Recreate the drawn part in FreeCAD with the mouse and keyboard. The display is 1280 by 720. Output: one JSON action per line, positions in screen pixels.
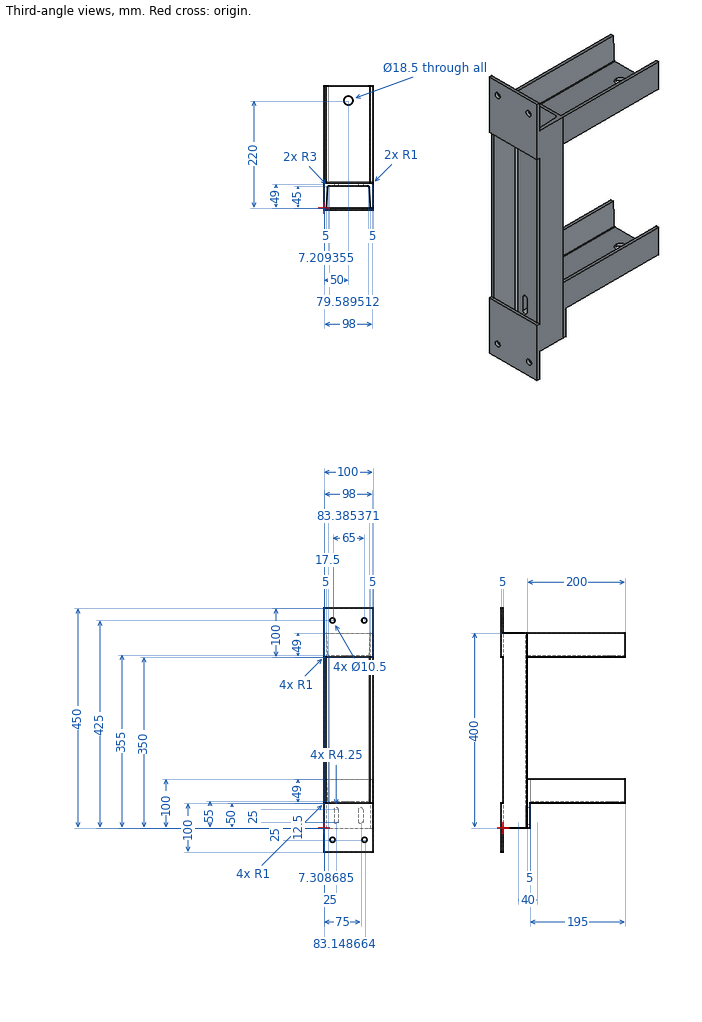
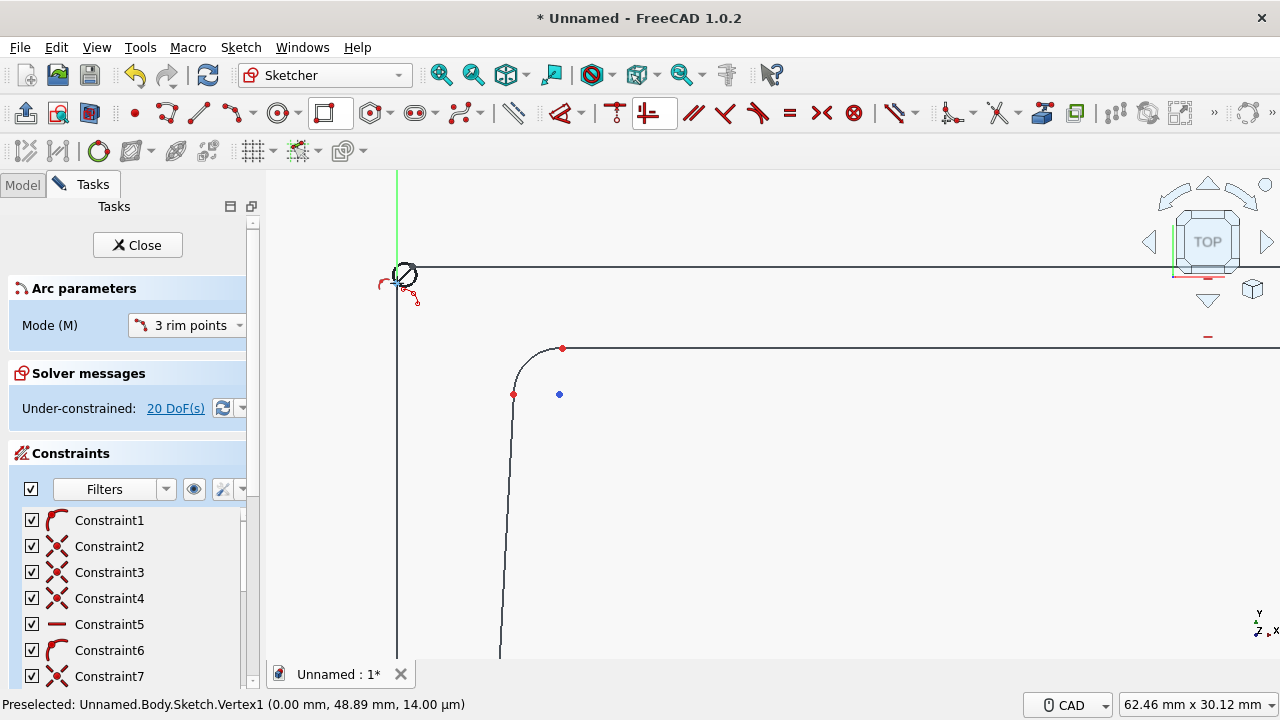
{"action": "scroll", "coordinate": [401, 270], "scroll_direction": "up", "scroll_amount": 7}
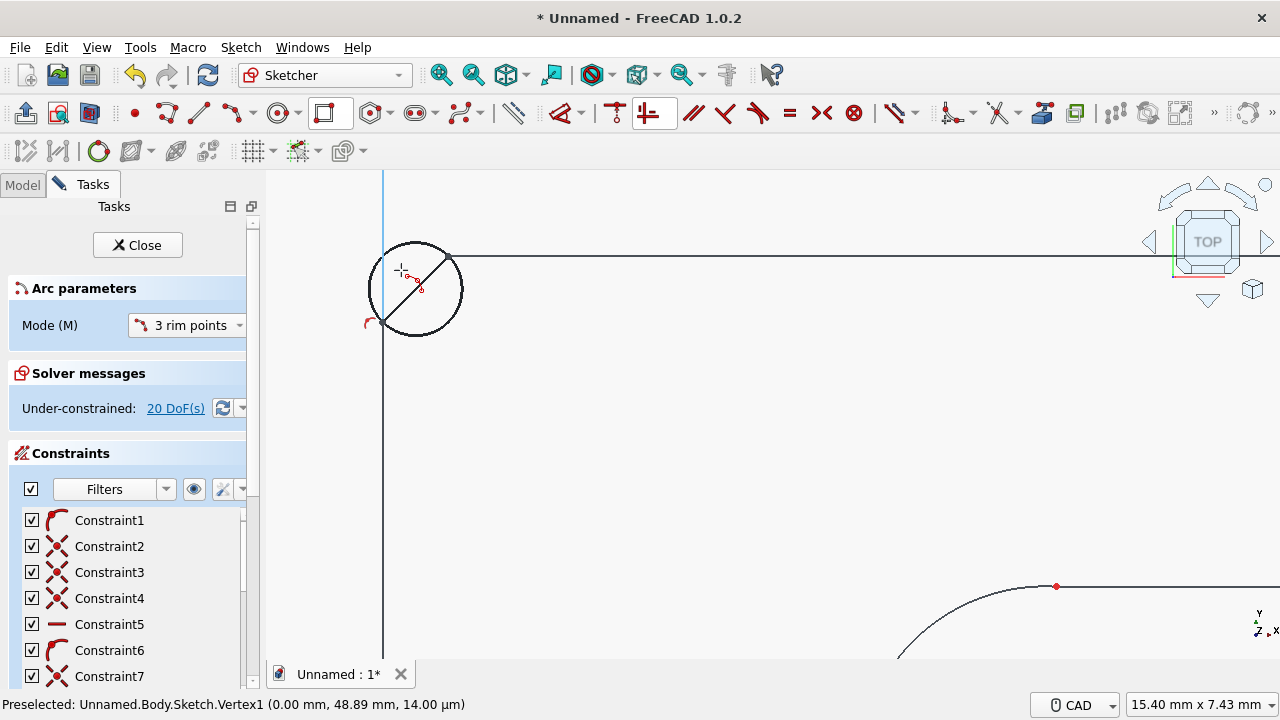
{"action": "left_click", "coordinate": [402, 268]}
{"action": "key", "text": "Escape"}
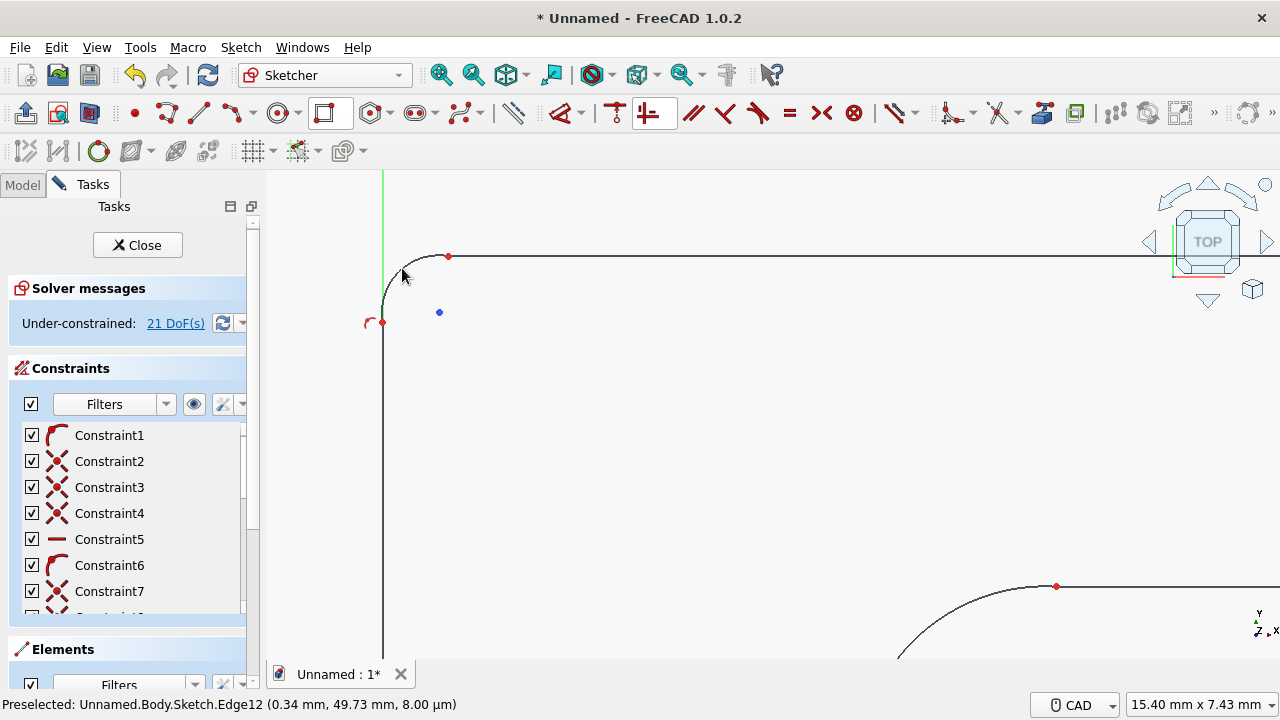
{"action": "scroll", "coordinate": [408, 267], "scroll_direction": "down", "scroll_amount": 12}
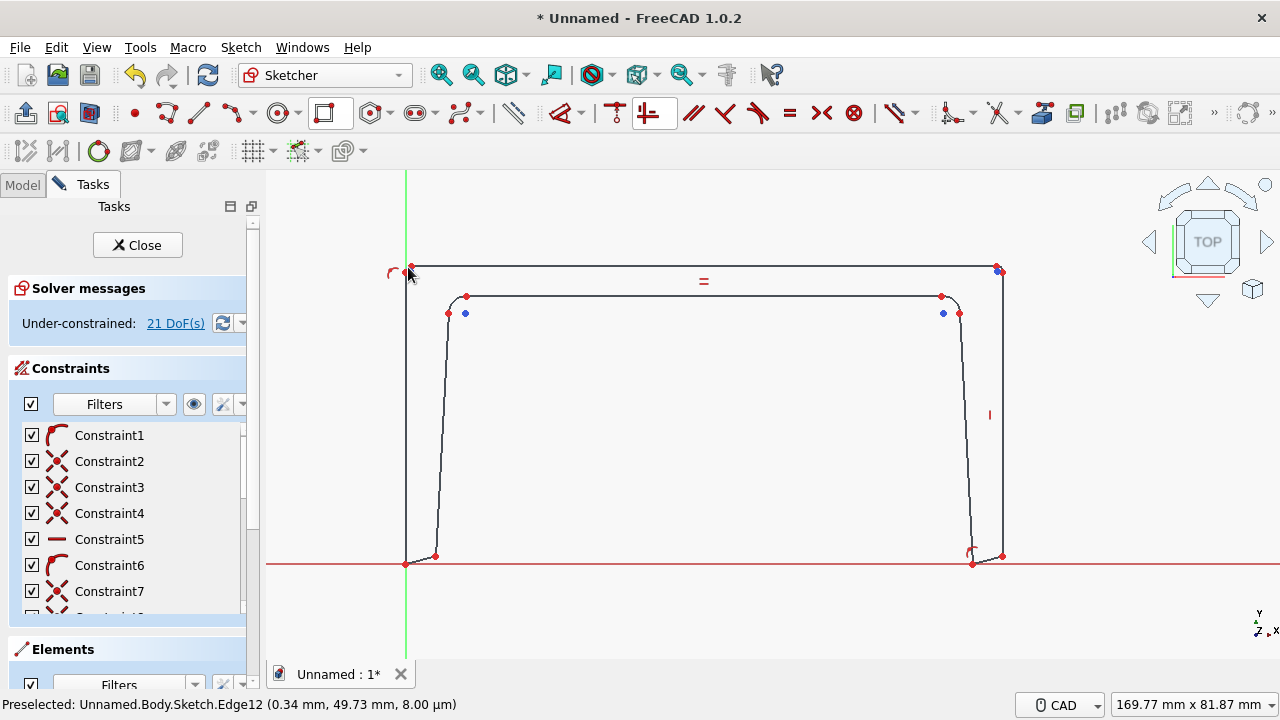
{"action": "left_click", "coordinate": [406, 360]}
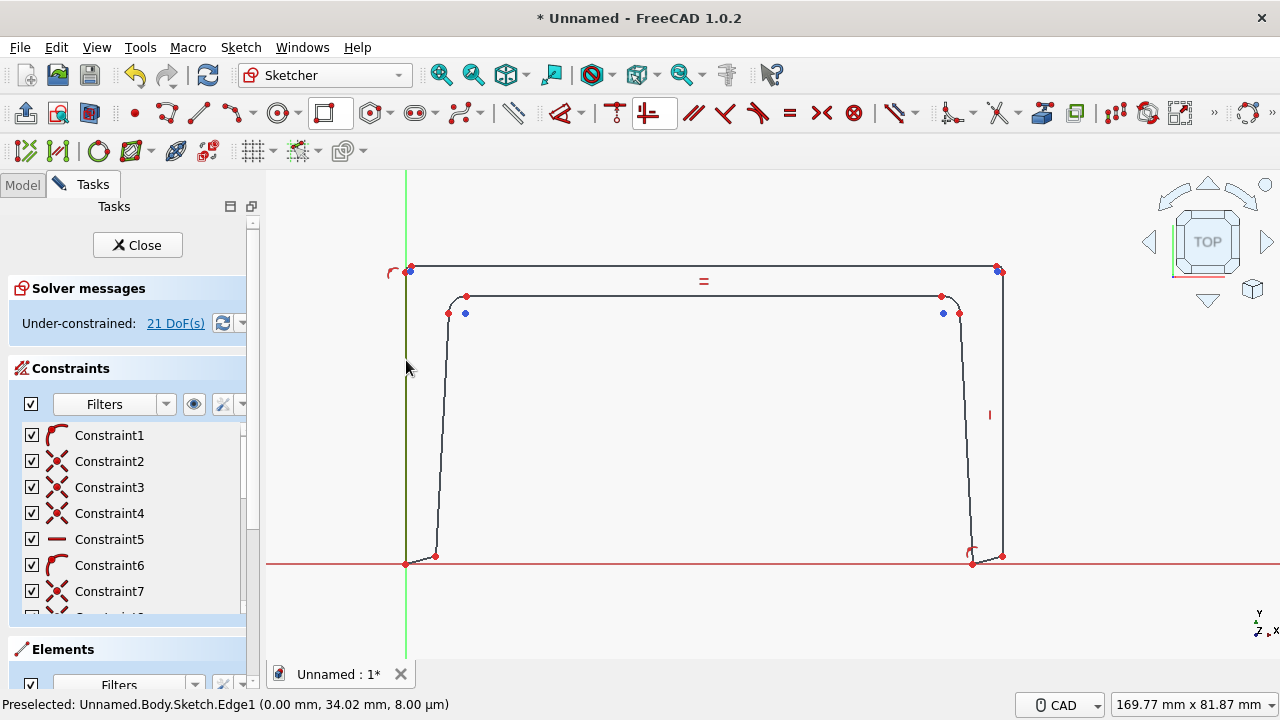
{"action": "scroll", "coordinate": [407, 268], "scroll_direction": "up", "scroll_amount": 6}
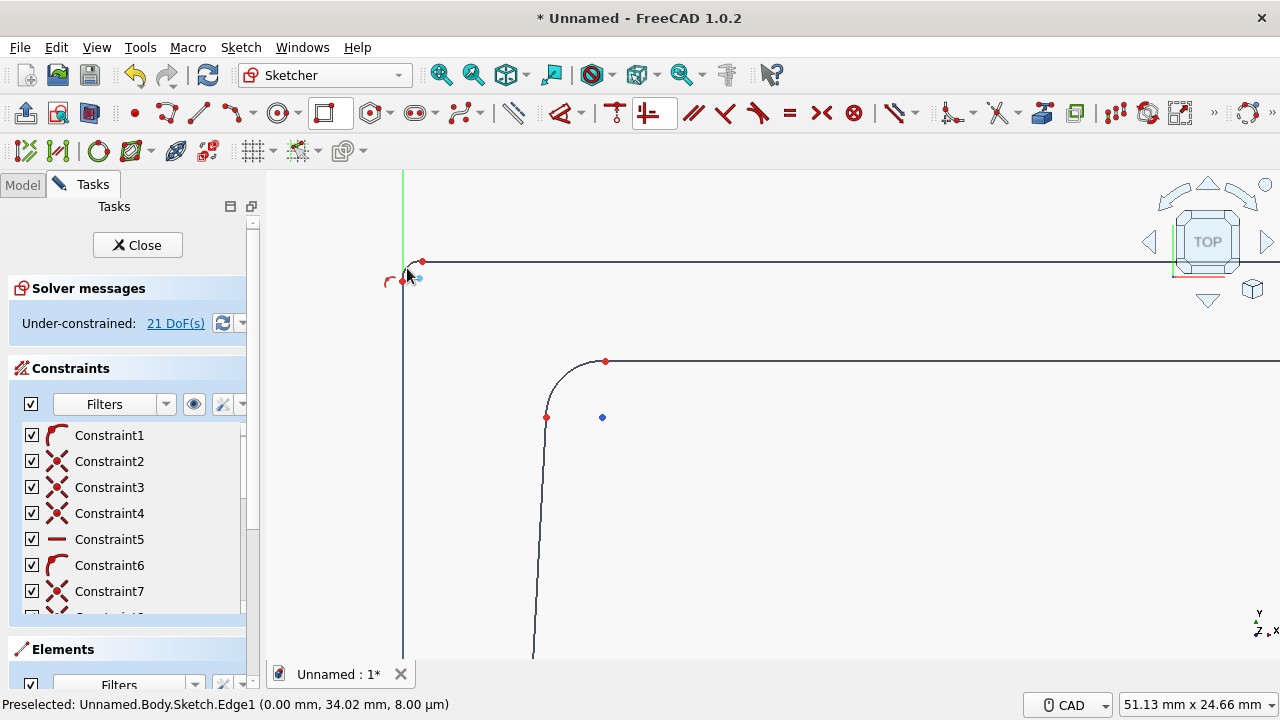
{"action": "left_click", "coordinate": [408, 266]}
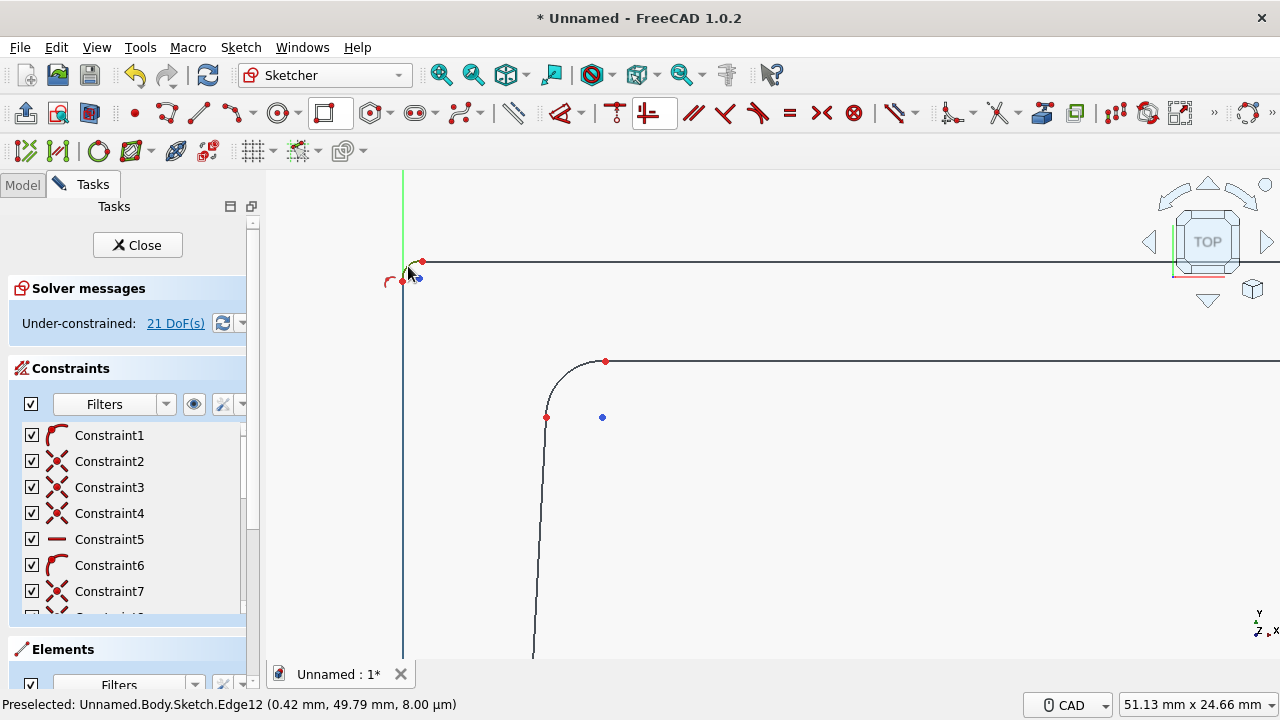
{"action": "left_click", "coordinate": [758, 114]}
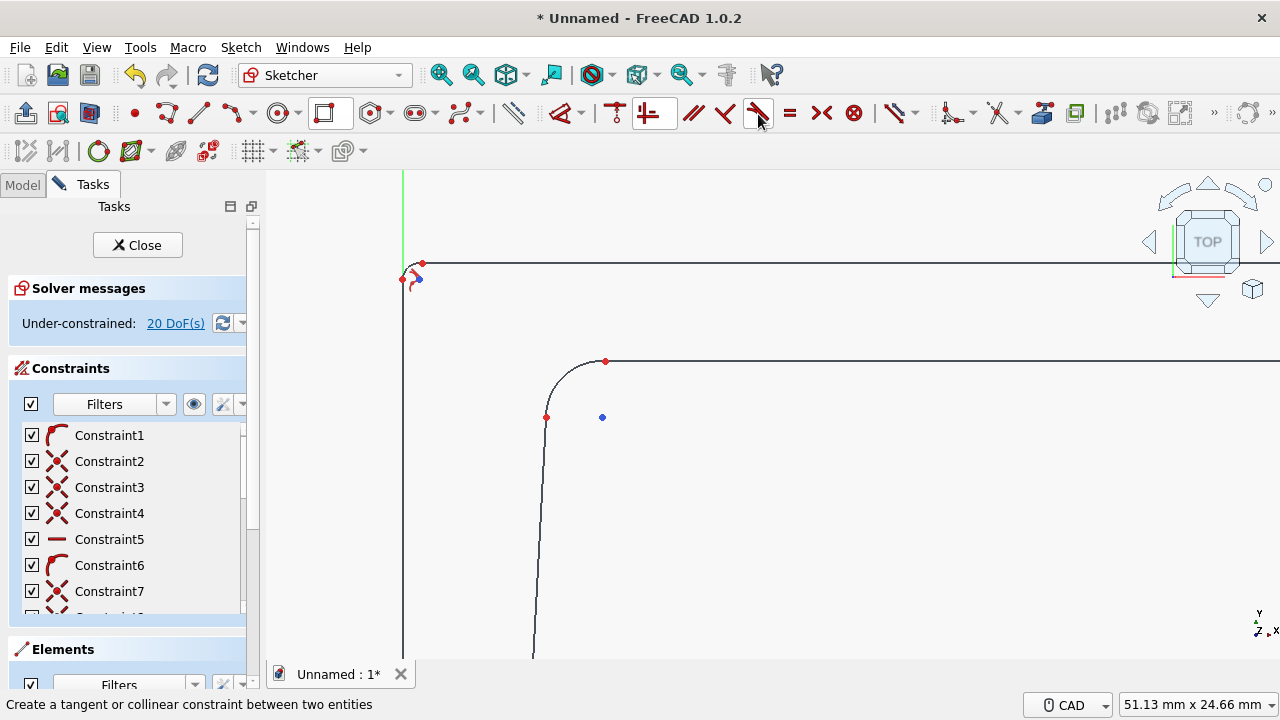
{"action": "left_click", "coordinate": [537, 579]}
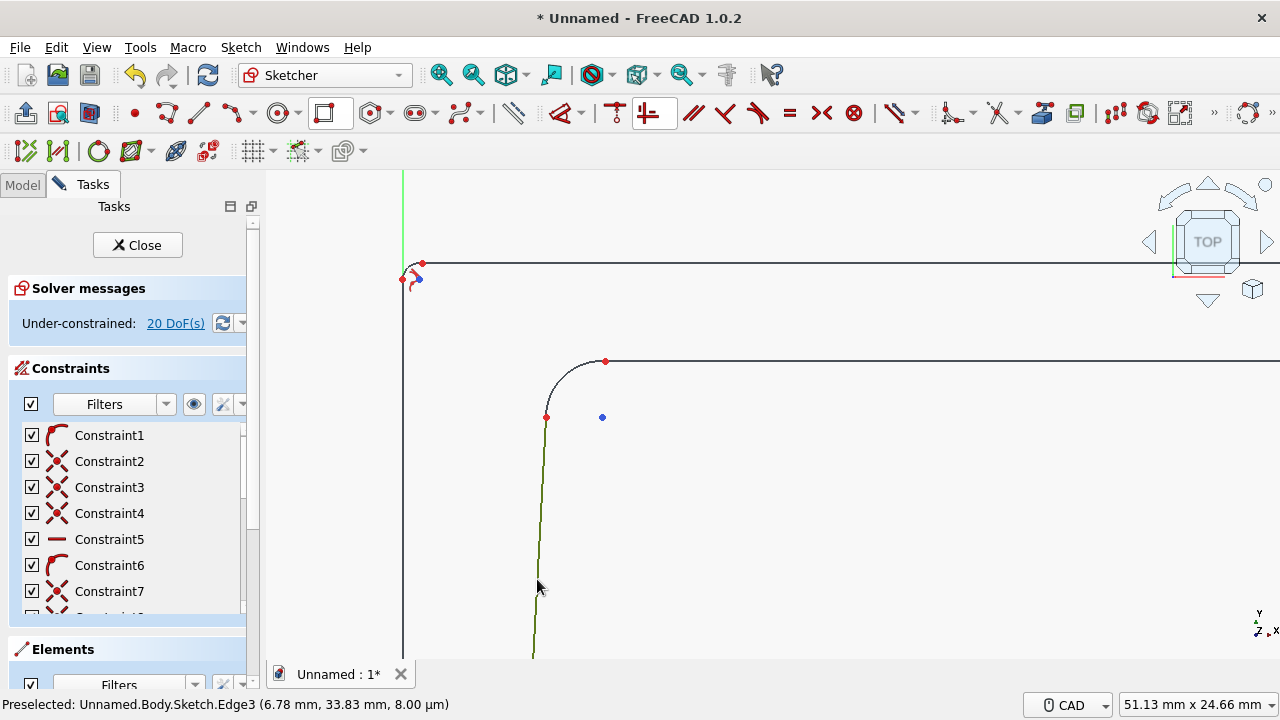
{"action": "left_click", "coordinate": [579, 366]}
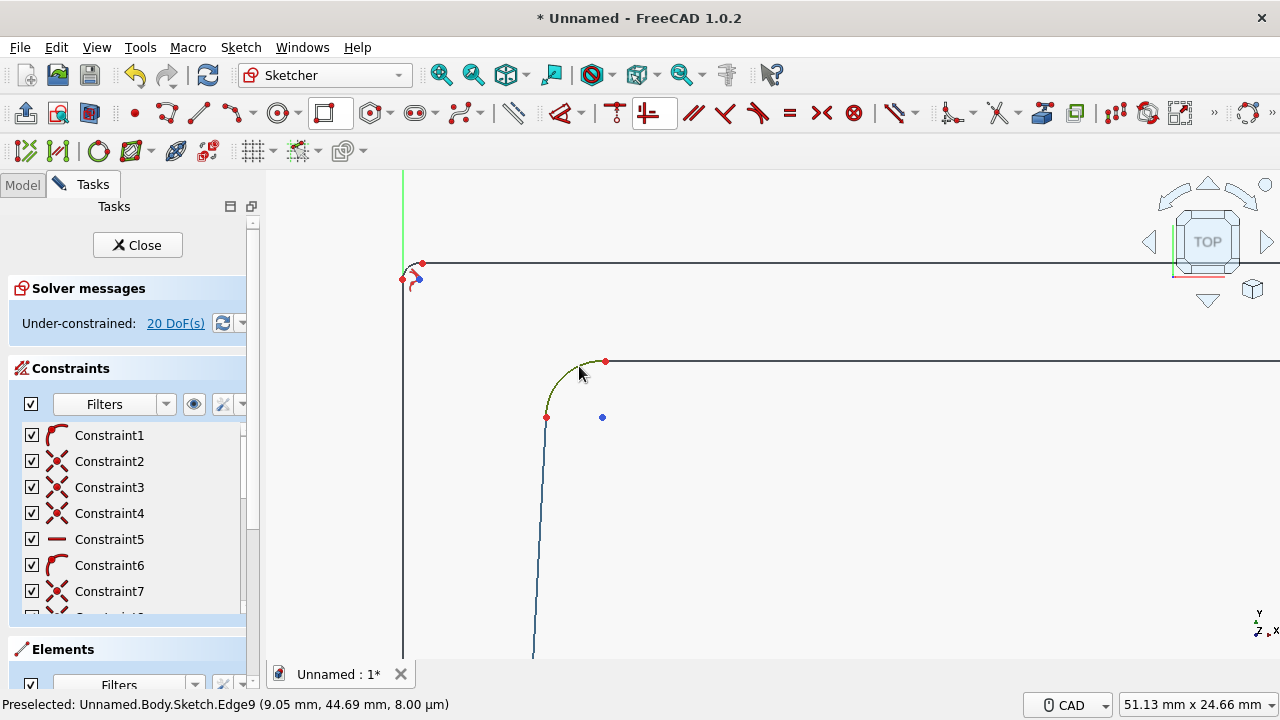
{"action": "left_click", "coordinate": [758, 114]}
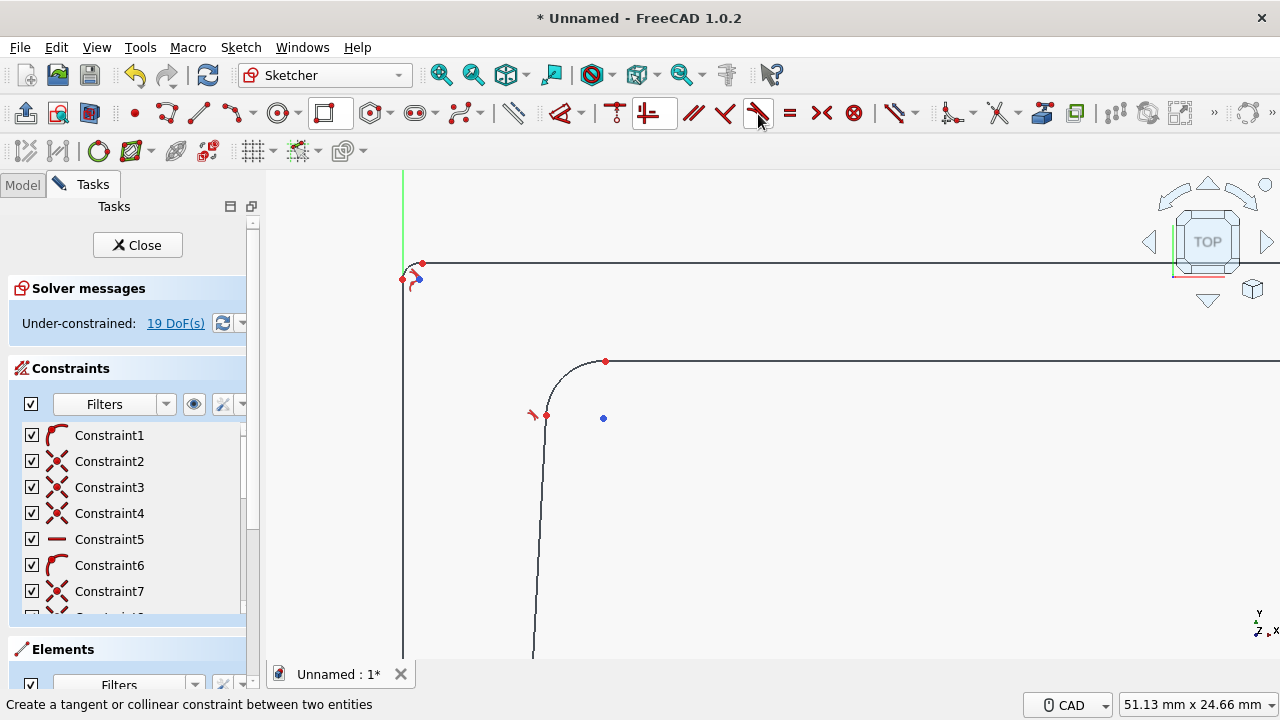
{"action": "left_click", "coordinate": [1079, 361]}